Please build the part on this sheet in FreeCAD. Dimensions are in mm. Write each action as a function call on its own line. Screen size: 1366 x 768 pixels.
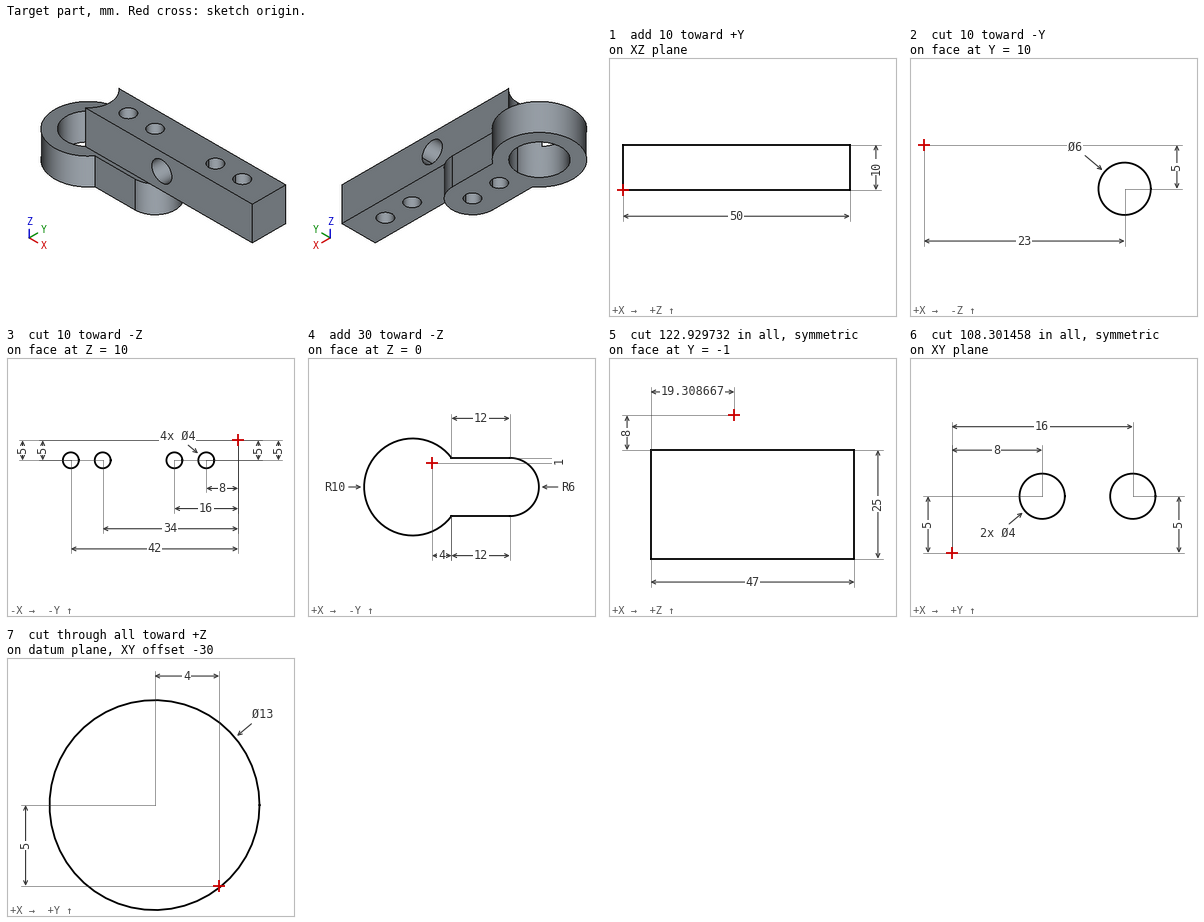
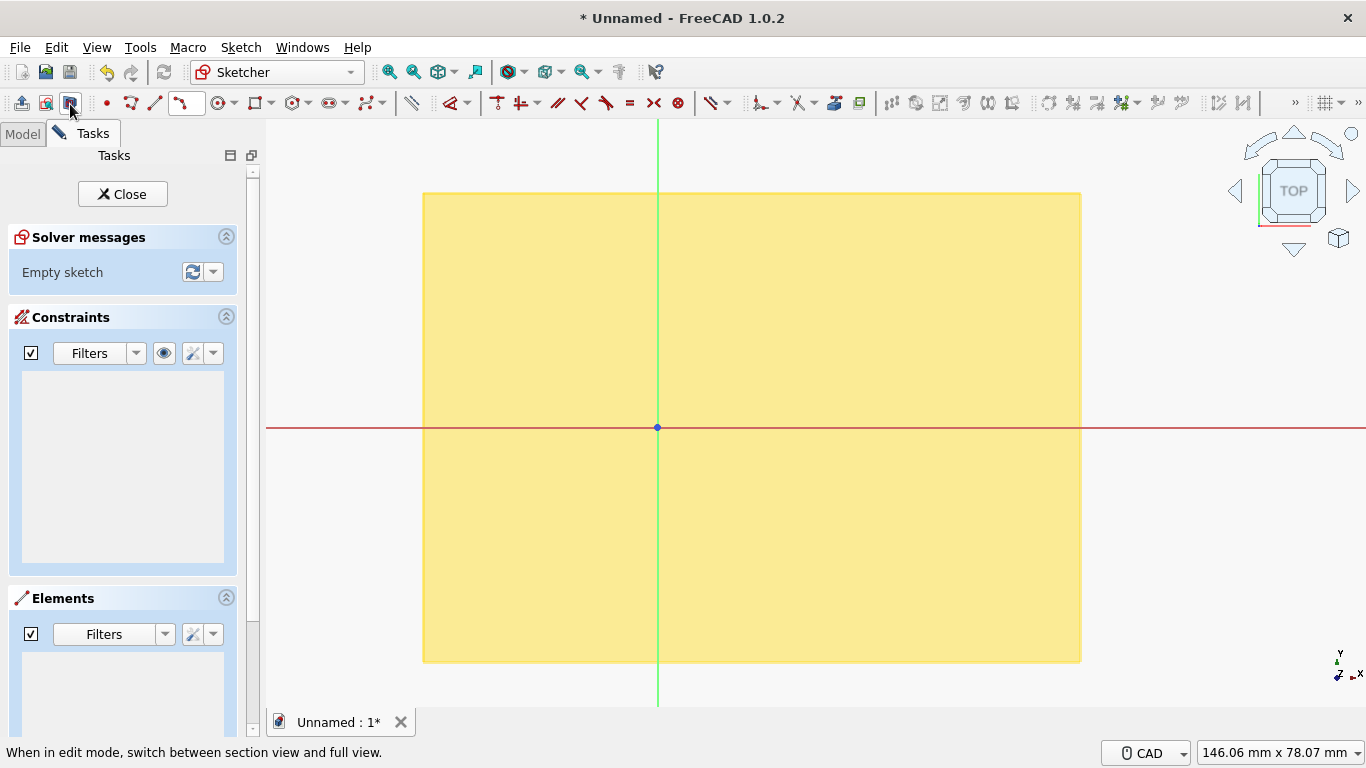
scroll(588, 383, up, 7)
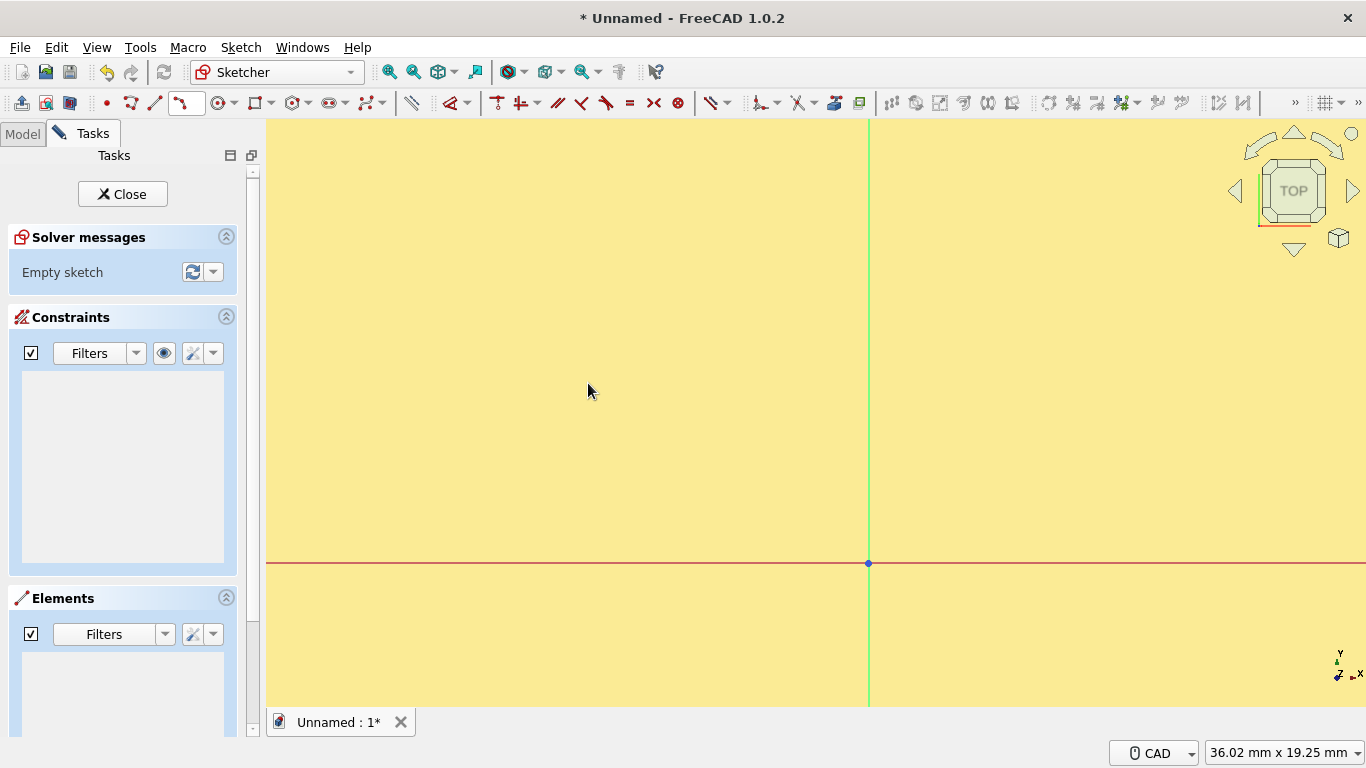
click(218, 104)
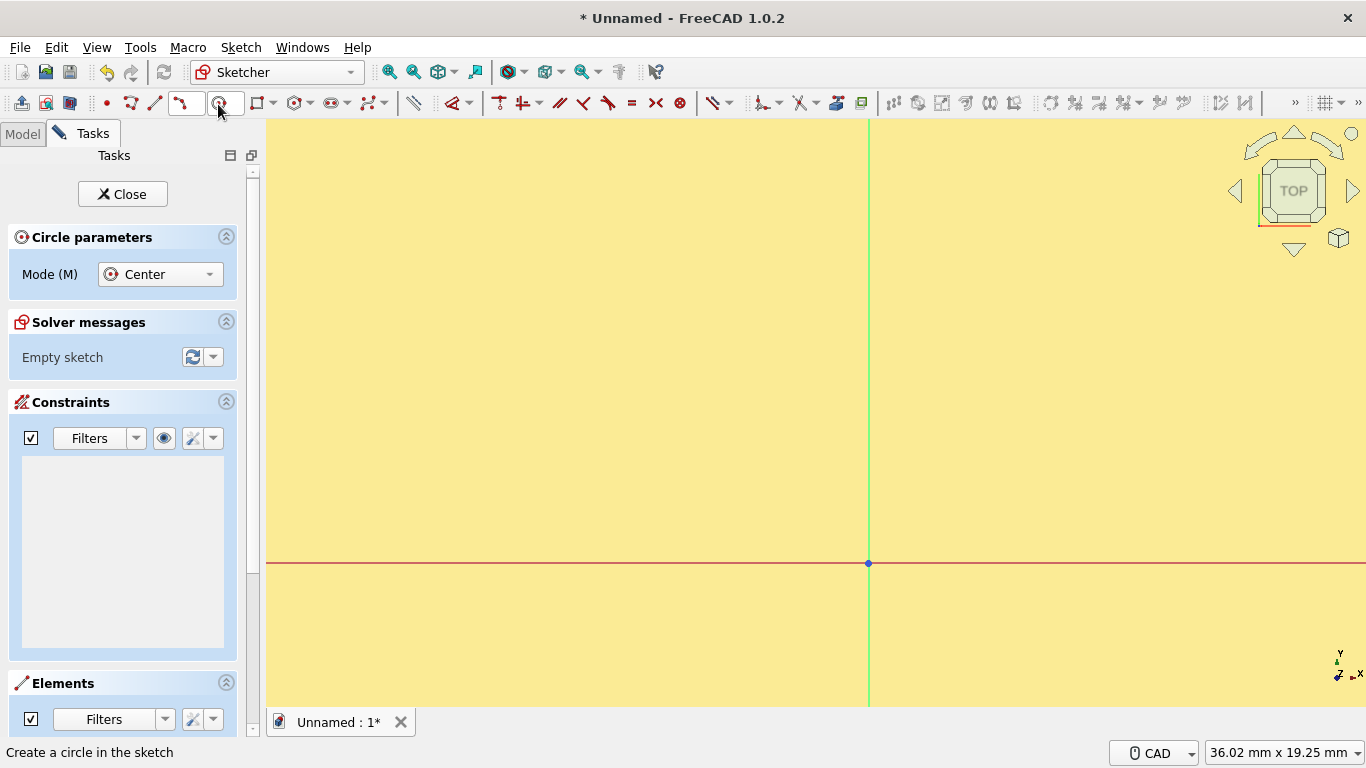
click(747, 410)
move(887, 270)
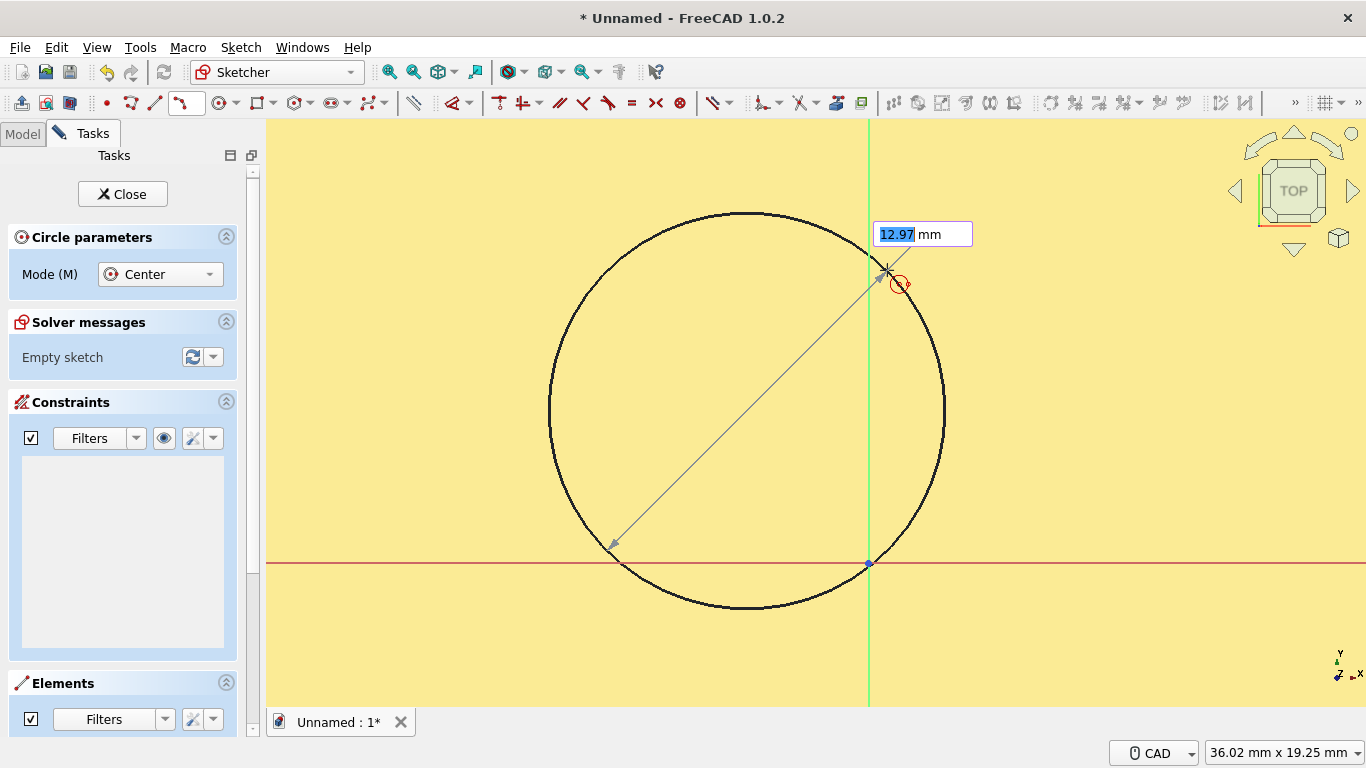
text(13)
key(Return)
key(Escape)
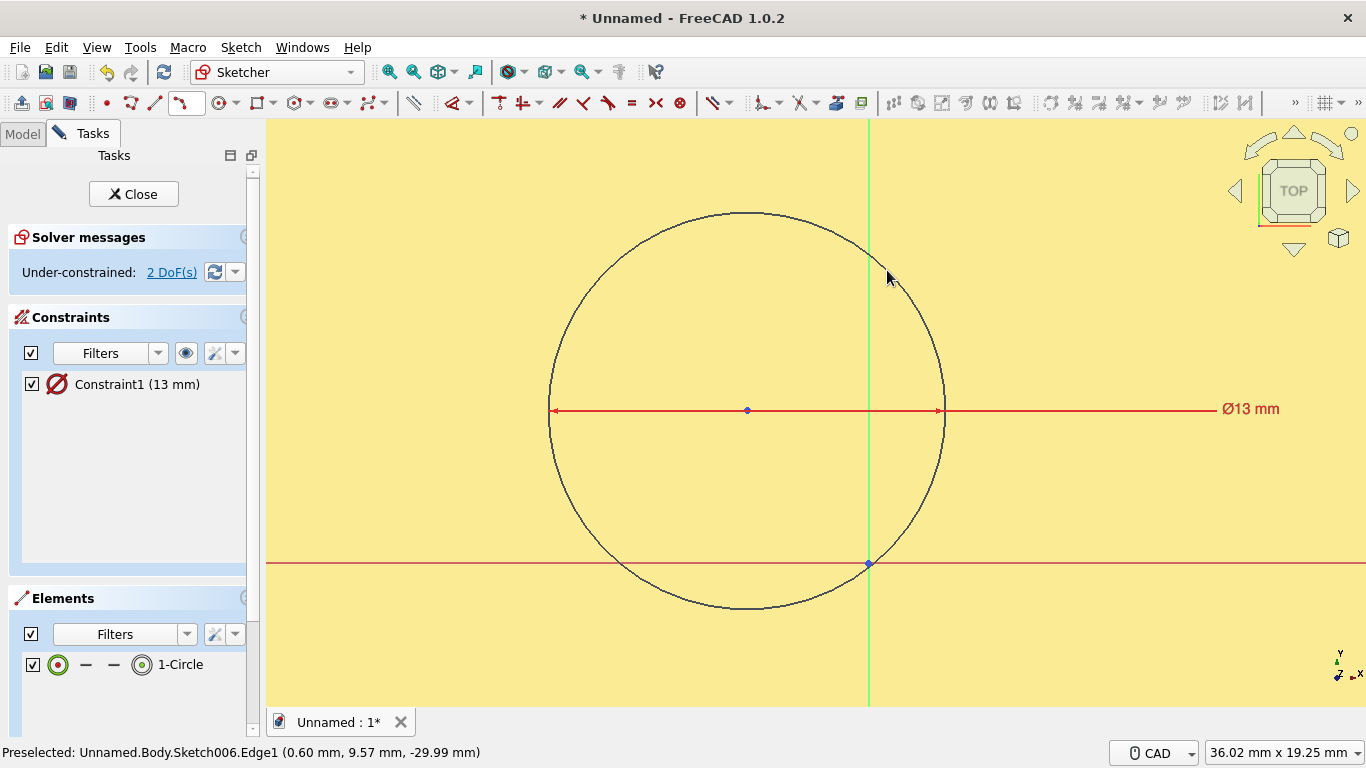
click(452, 104)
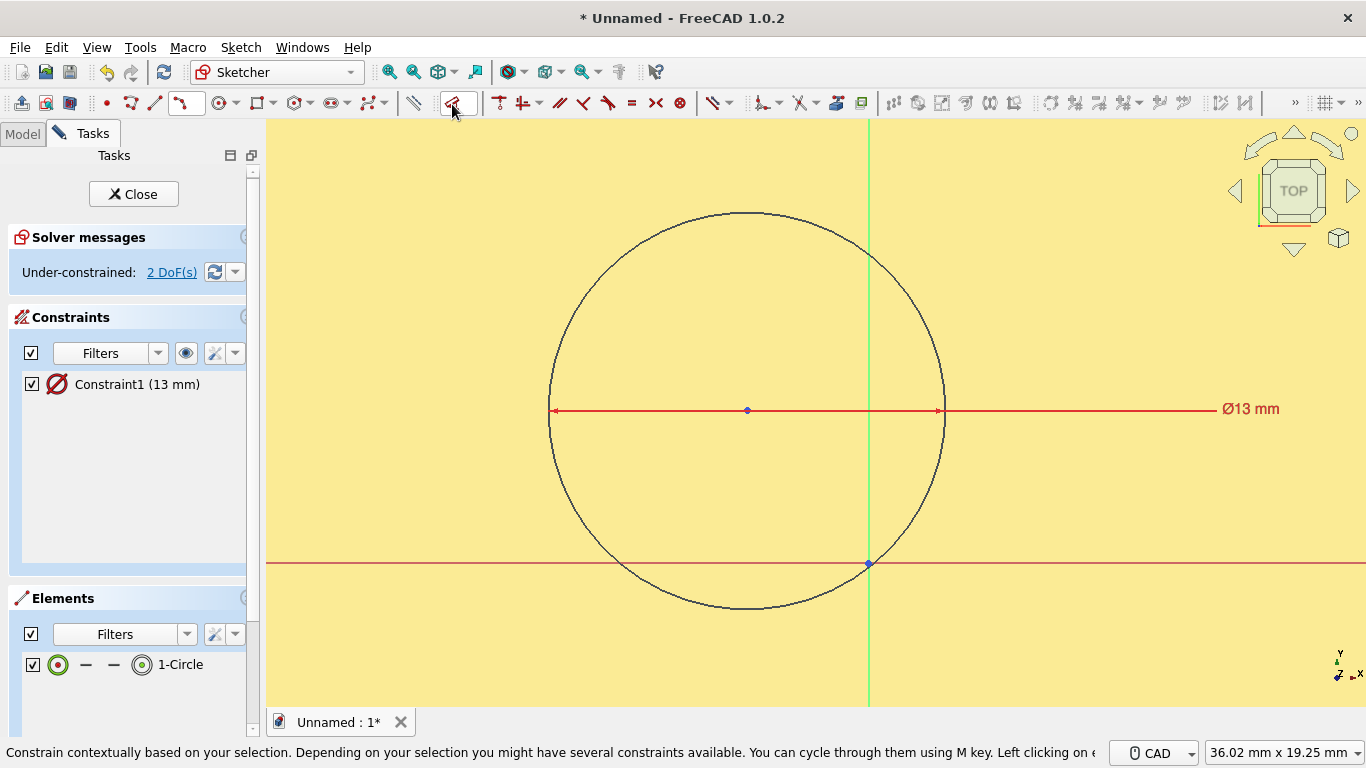
click(747, 411)
click(851, 597)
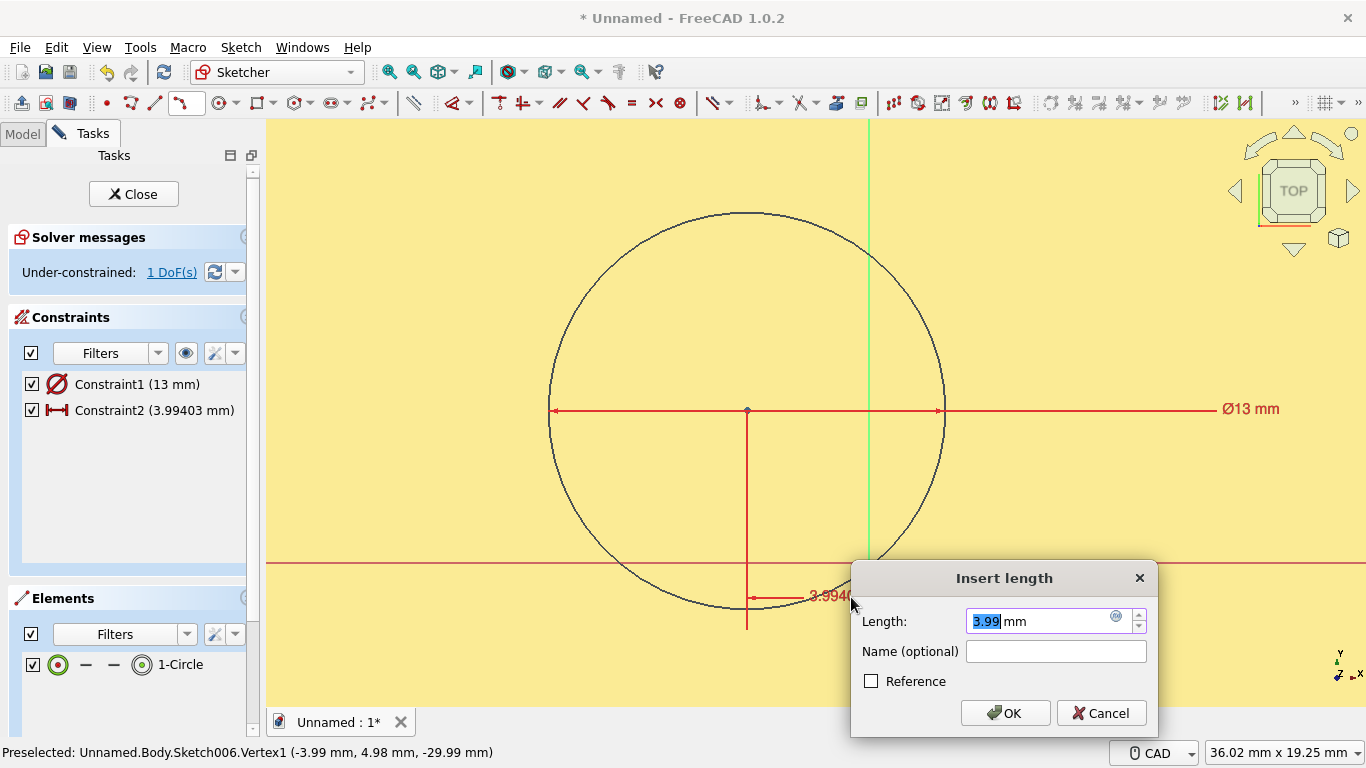
text(4)
key(Return)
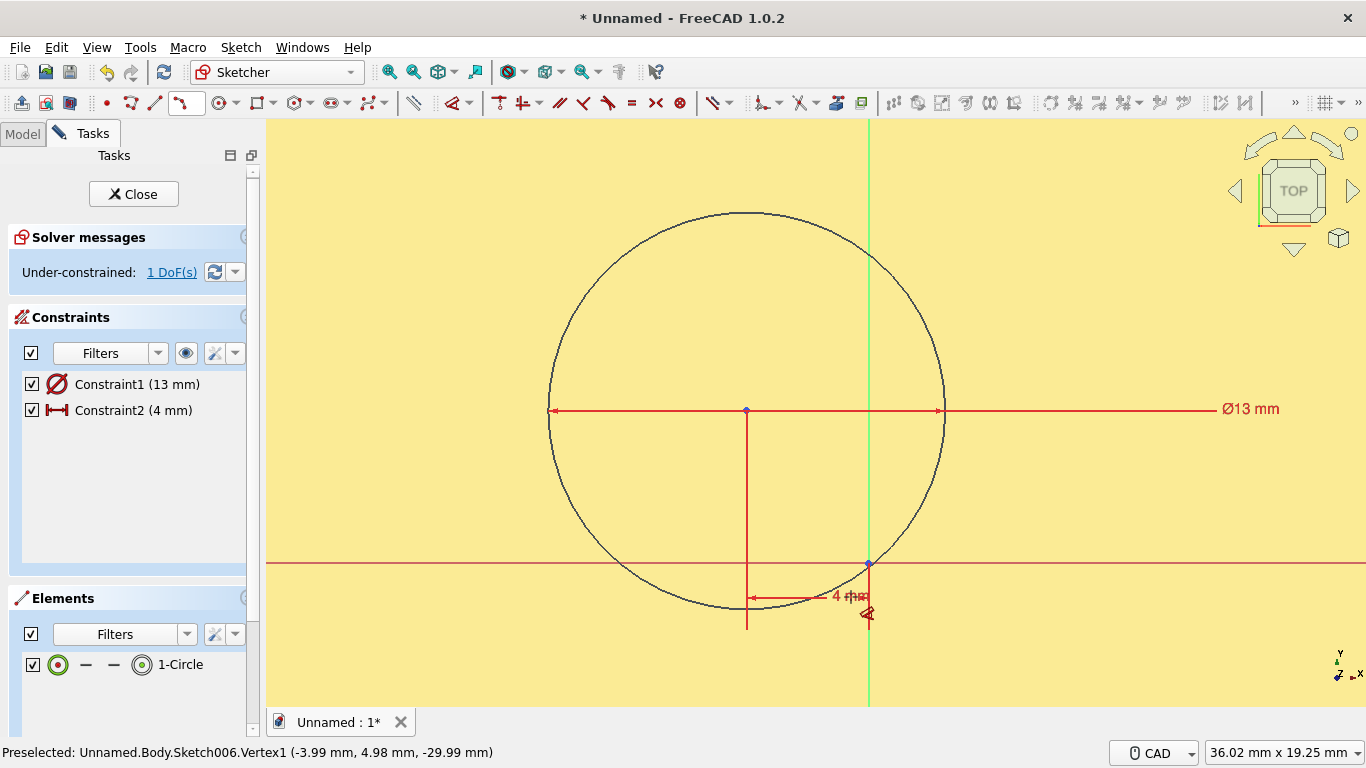
click(747, 411)
click(903, 487)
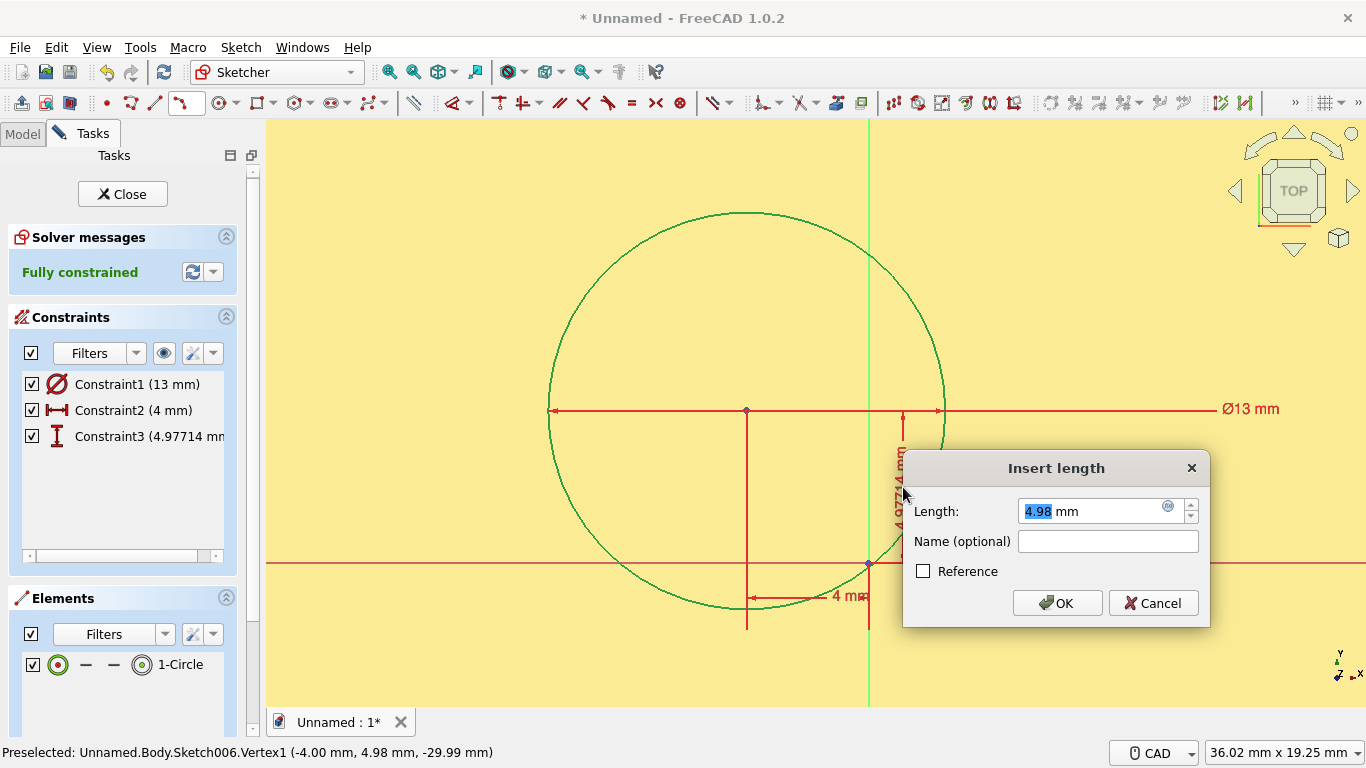
text(5)
key(Return)
key(Escape)